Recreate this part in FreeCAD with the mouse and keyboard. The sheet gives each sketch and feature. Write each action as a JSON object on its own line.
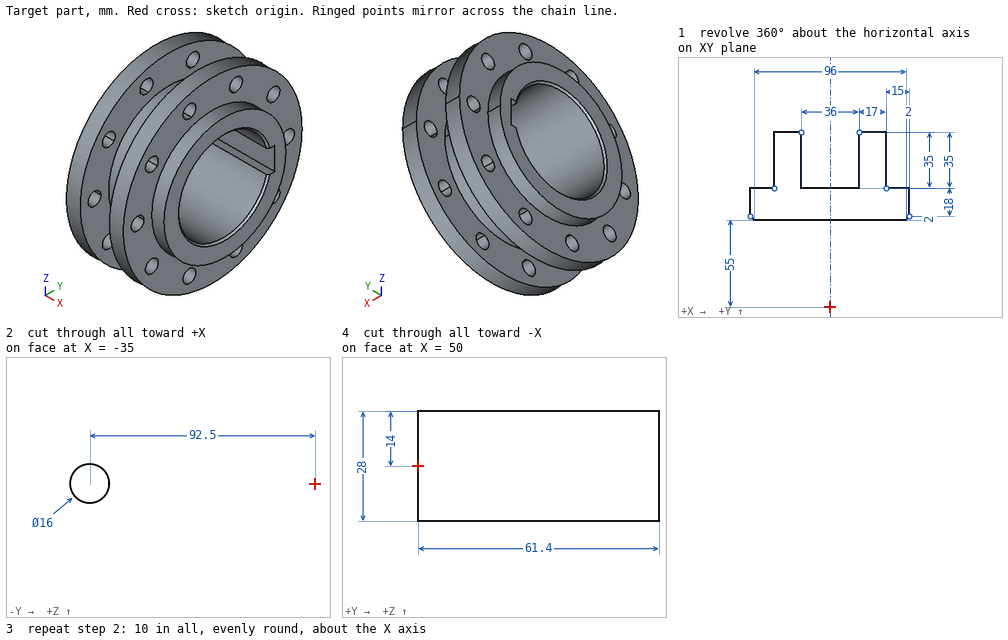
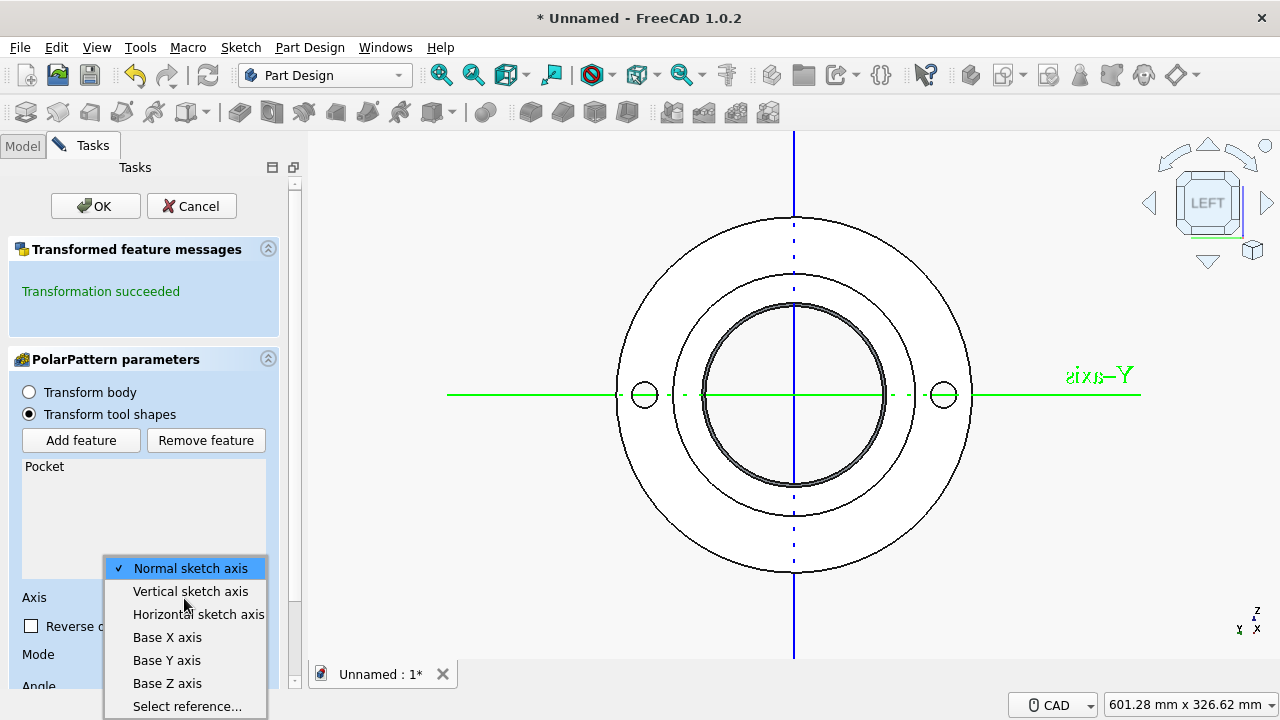
{"action": "left_click", "coordinate": [184, 638]}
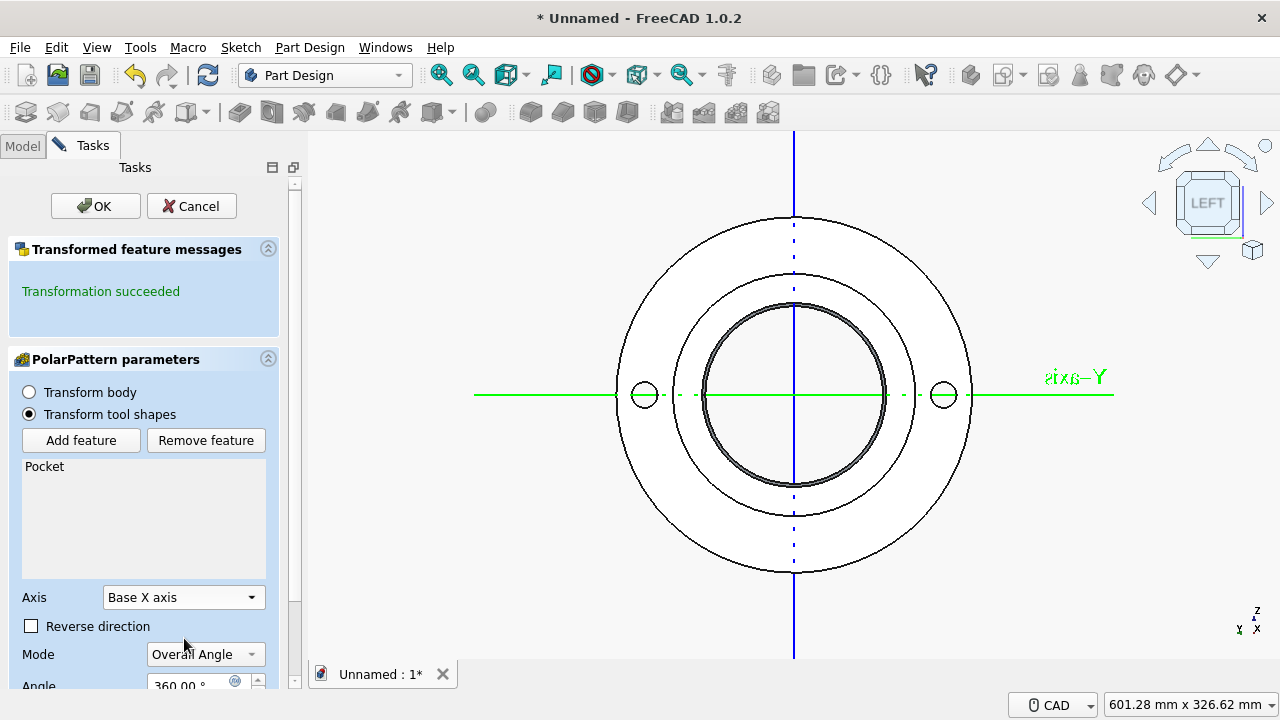
{"action": "scroll", "coordinate": [295, 432], "scroll_direction": "down", "scroll_amount": 2}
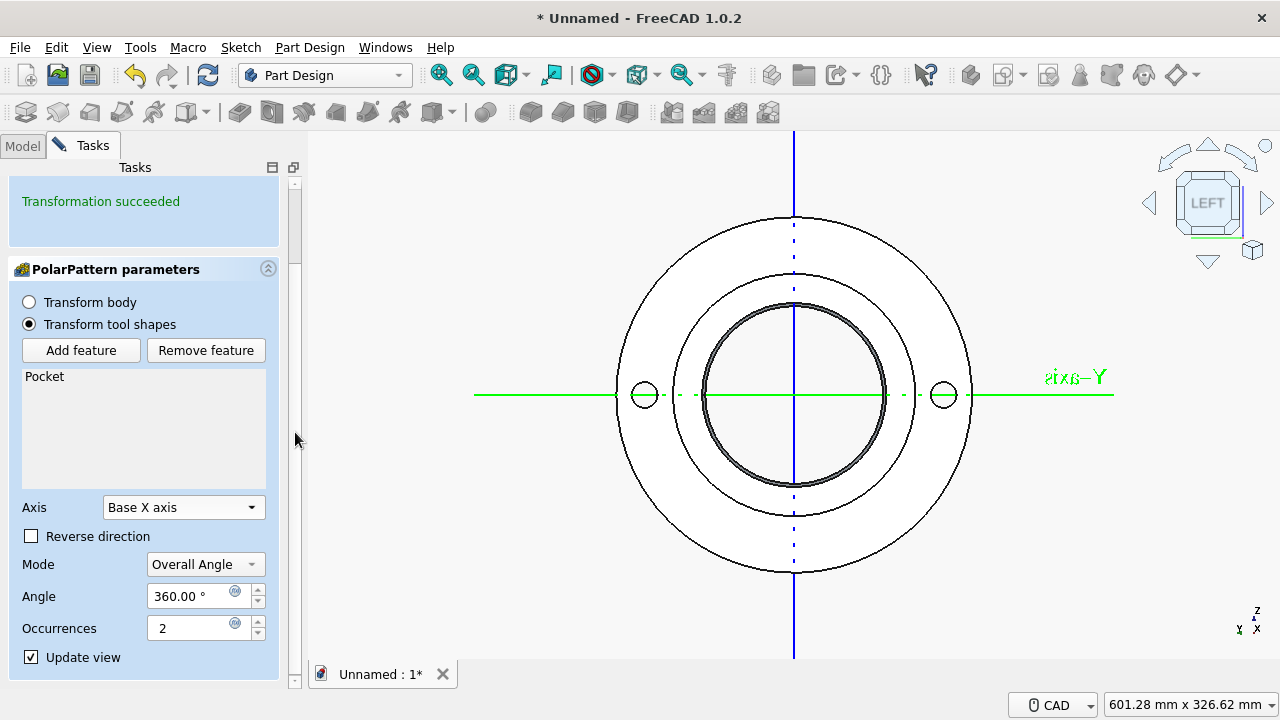
{"action": "triple_click", "coordinate": [198, 628]}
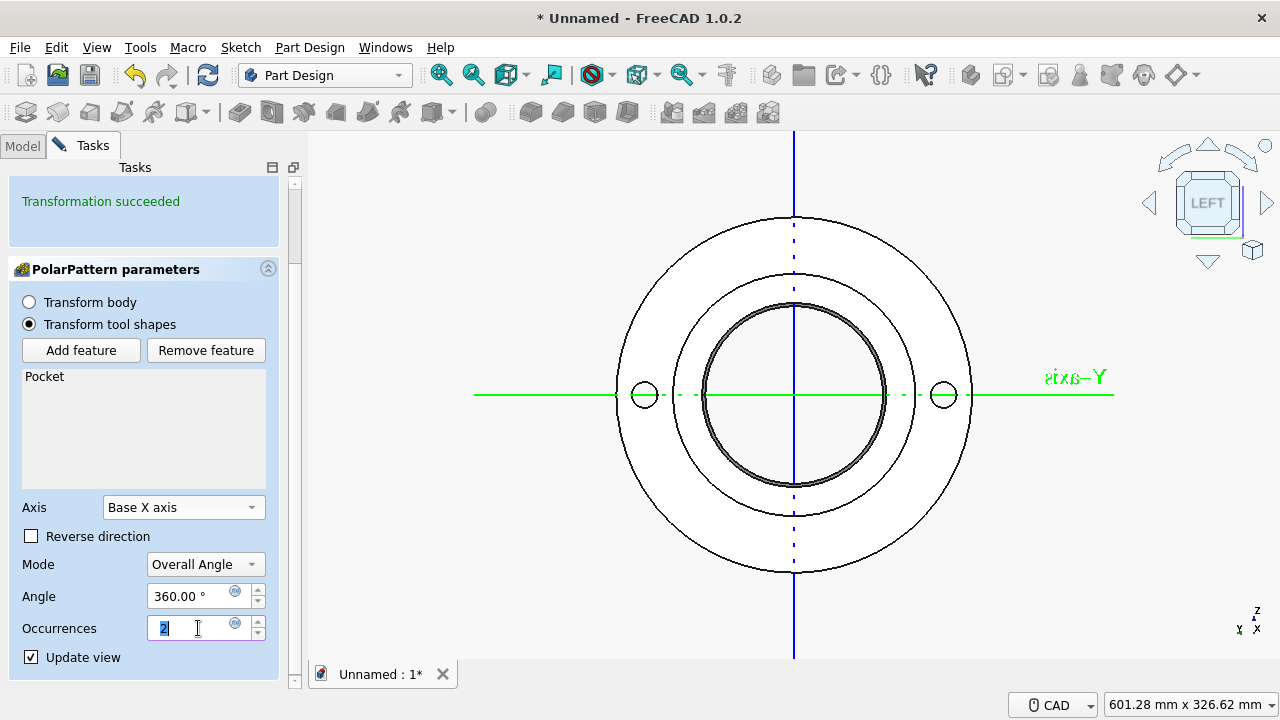
{"action": "type", "text": "10"}
{"action": "key", "text": "Tab"}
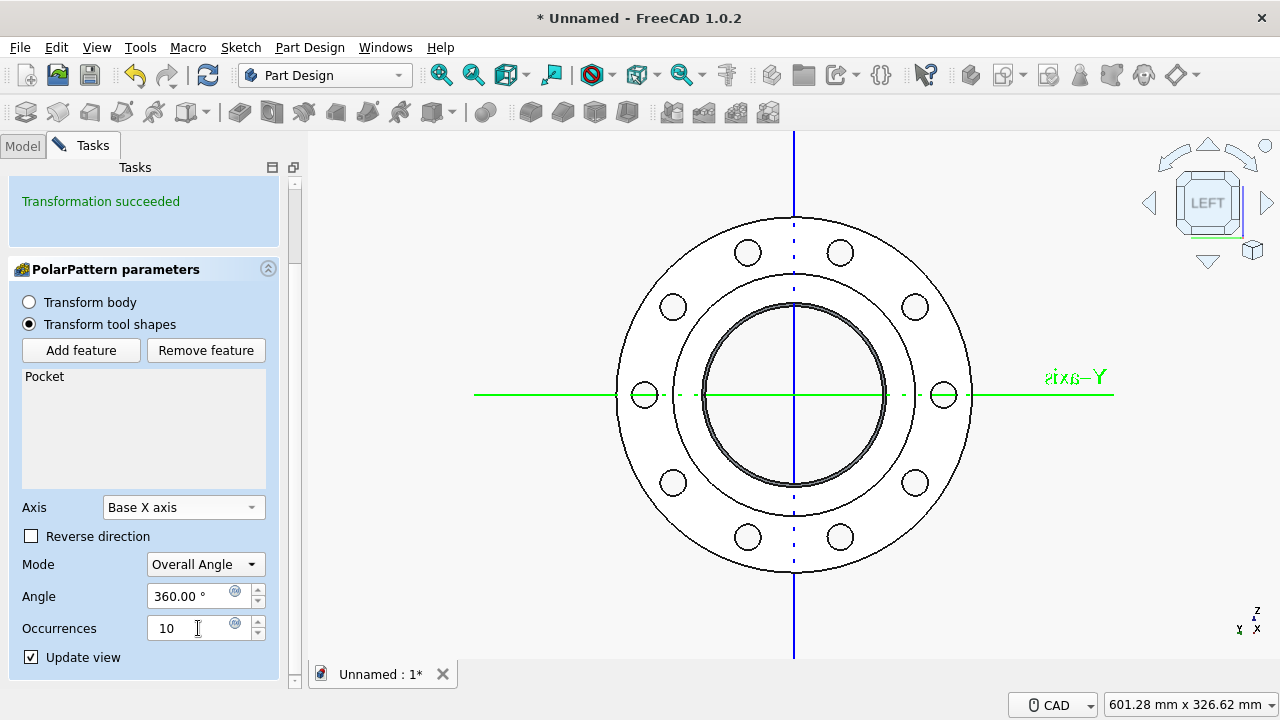
{"action": "scroll", "coordinate": [295, 432], "scroll_direction": "up", "scroll_amount": 3}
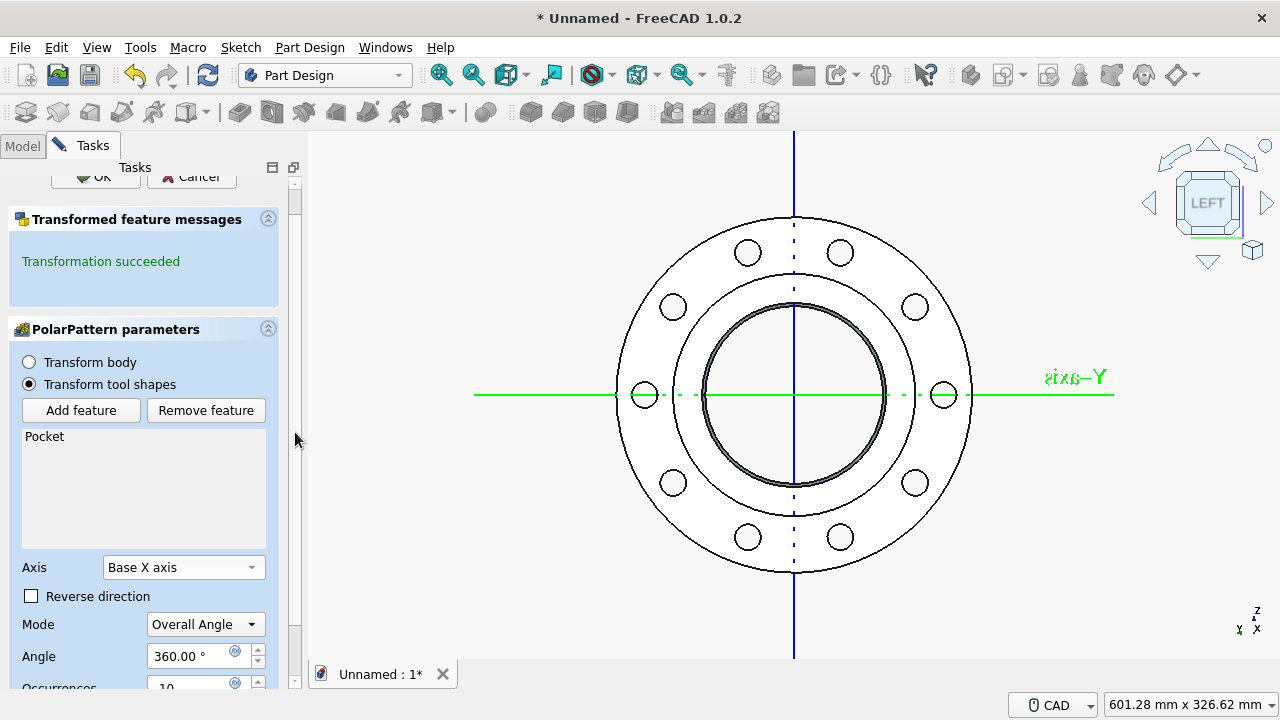
{"action": "left_click", "coordinate": [96, 206]}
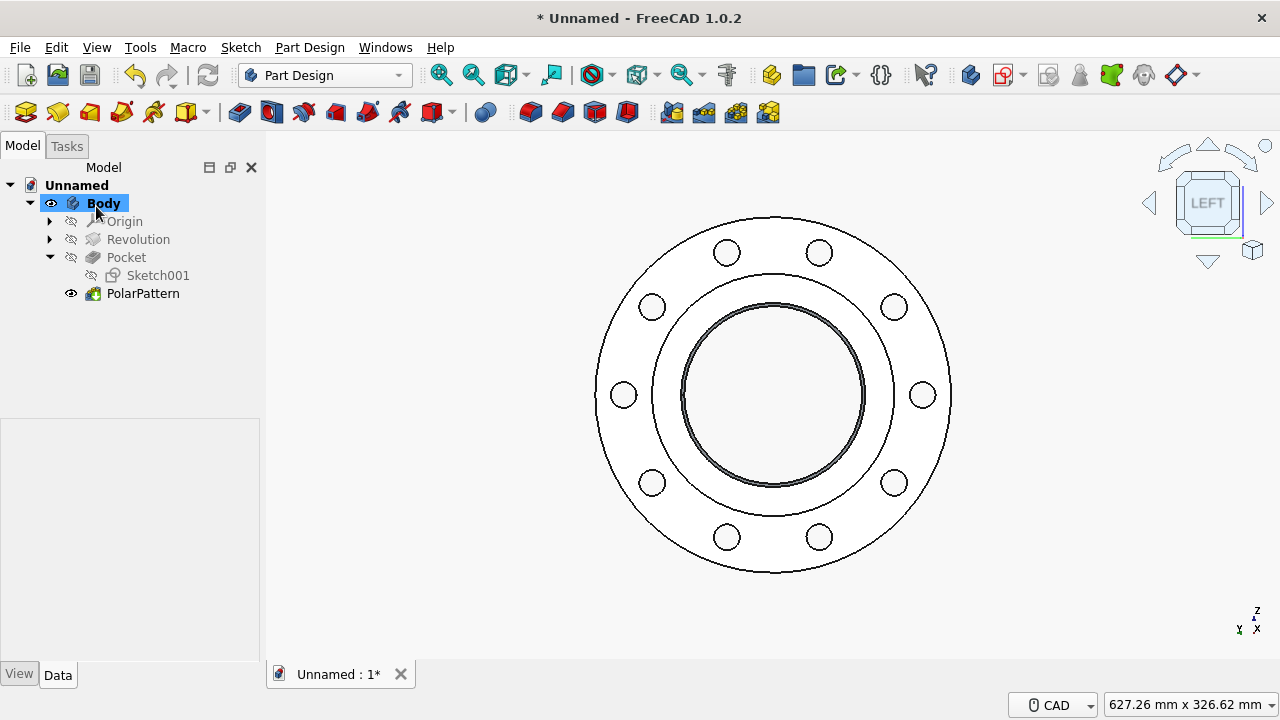
{"action": "key", "text": "0"}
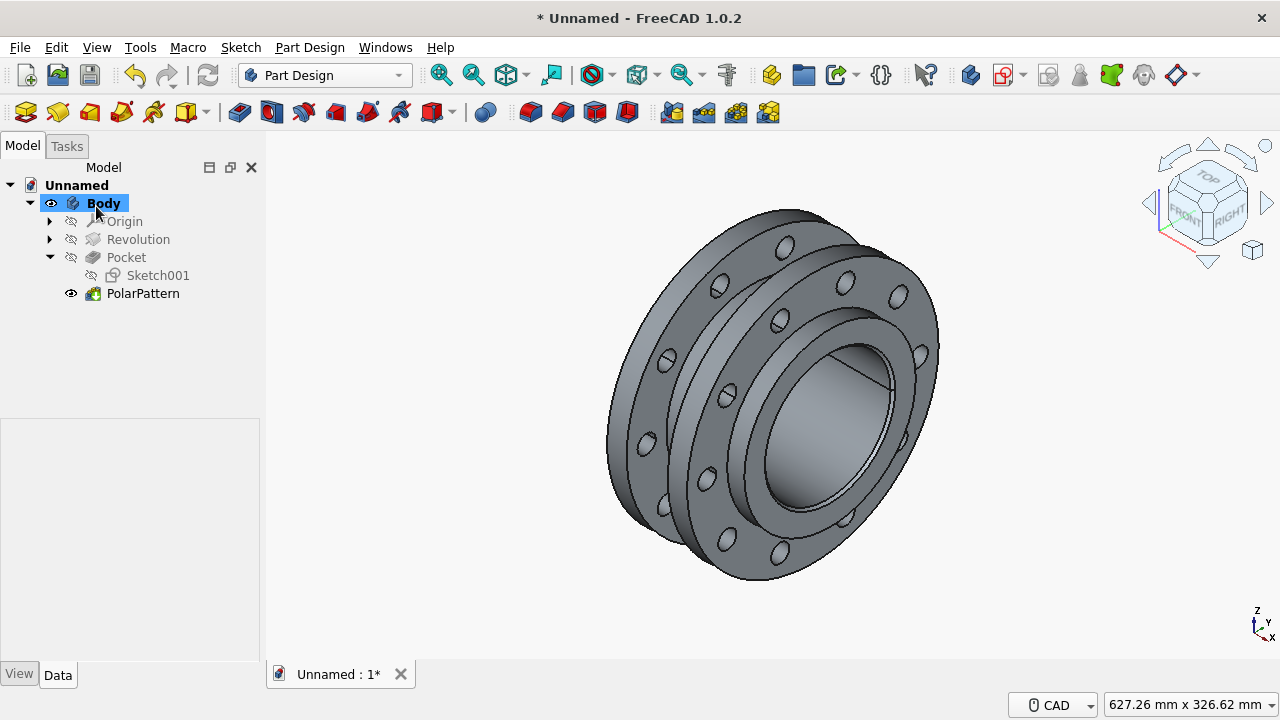
{"action": "left_click", "coordinate": [904, 385]}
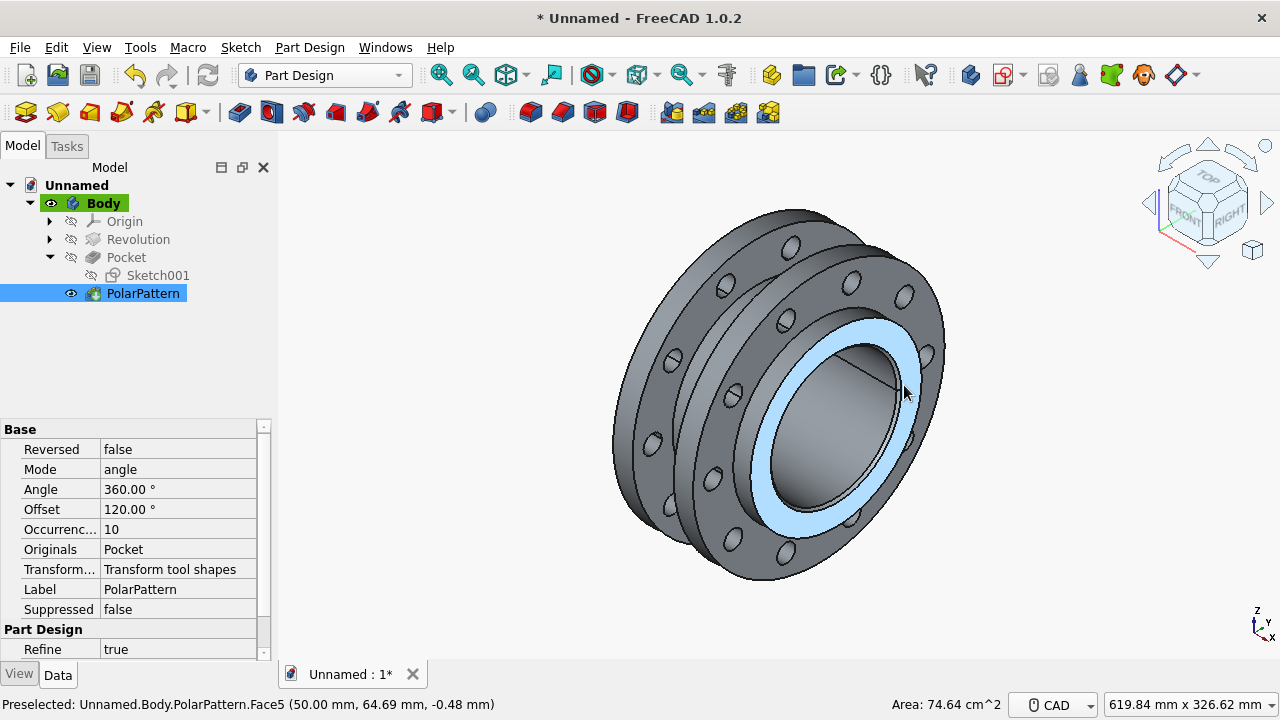
{"action": "left_click", "coordinate": [1004, 76]}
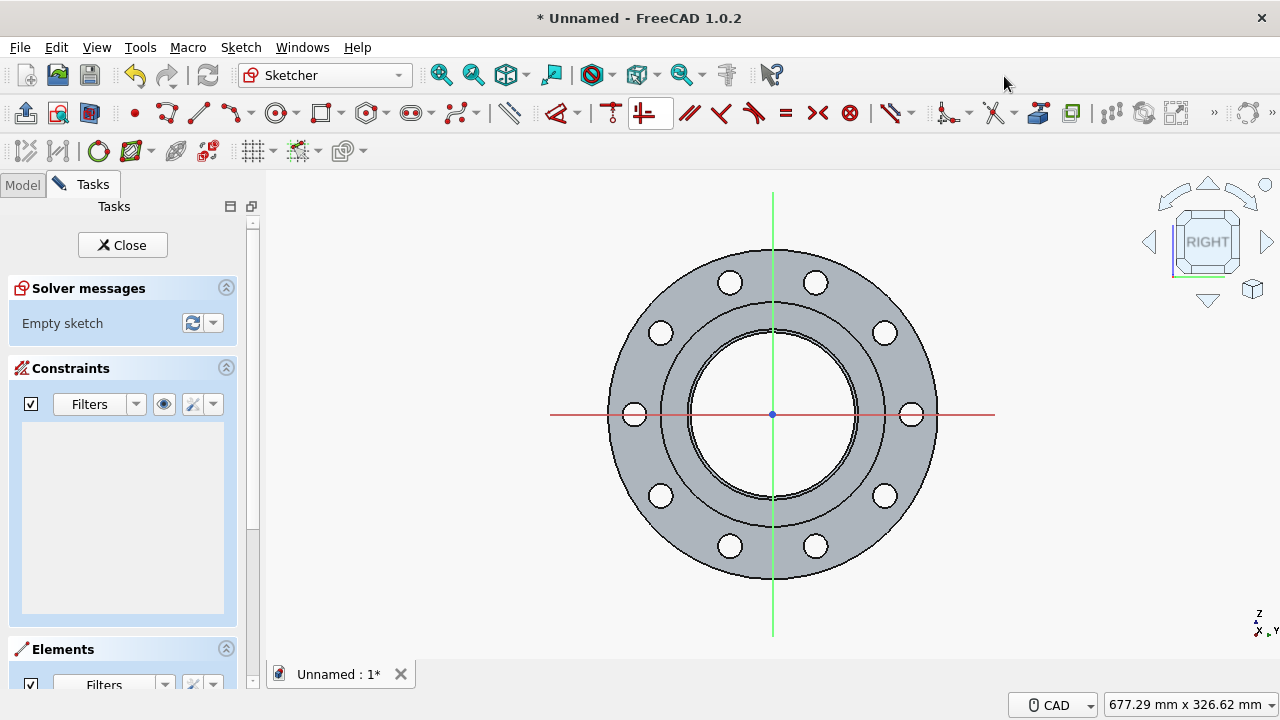
{"action": "scroll", "coordinate": [841, 415], "scroll_direction": "up", "scroll_amount": 9}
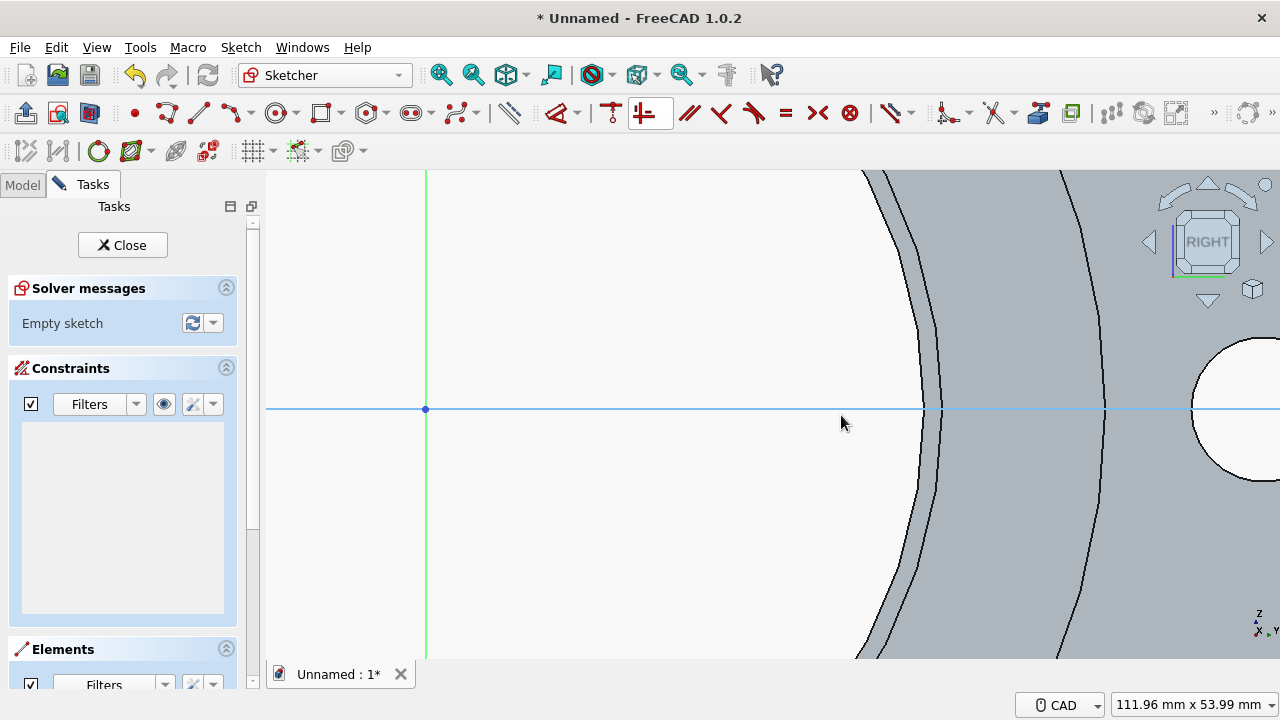
{"action": "left_click", "coordinate": [322, 114]}